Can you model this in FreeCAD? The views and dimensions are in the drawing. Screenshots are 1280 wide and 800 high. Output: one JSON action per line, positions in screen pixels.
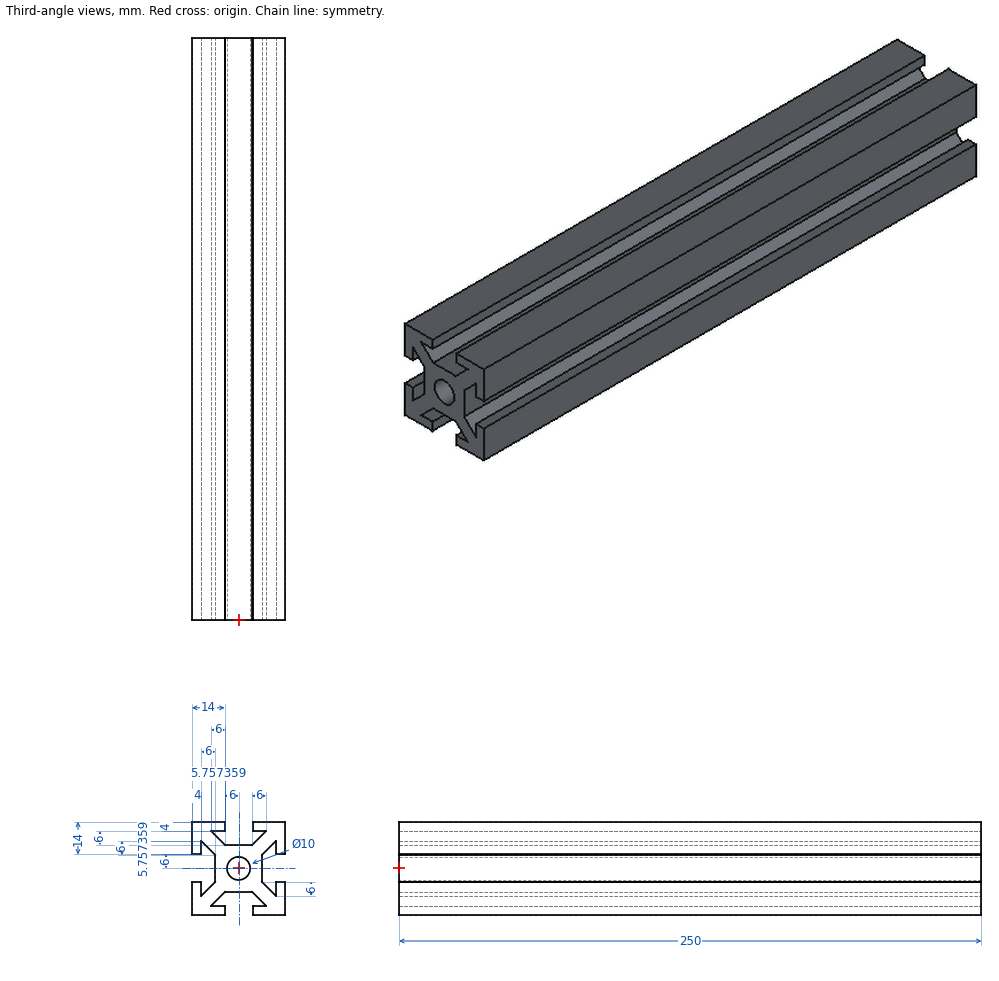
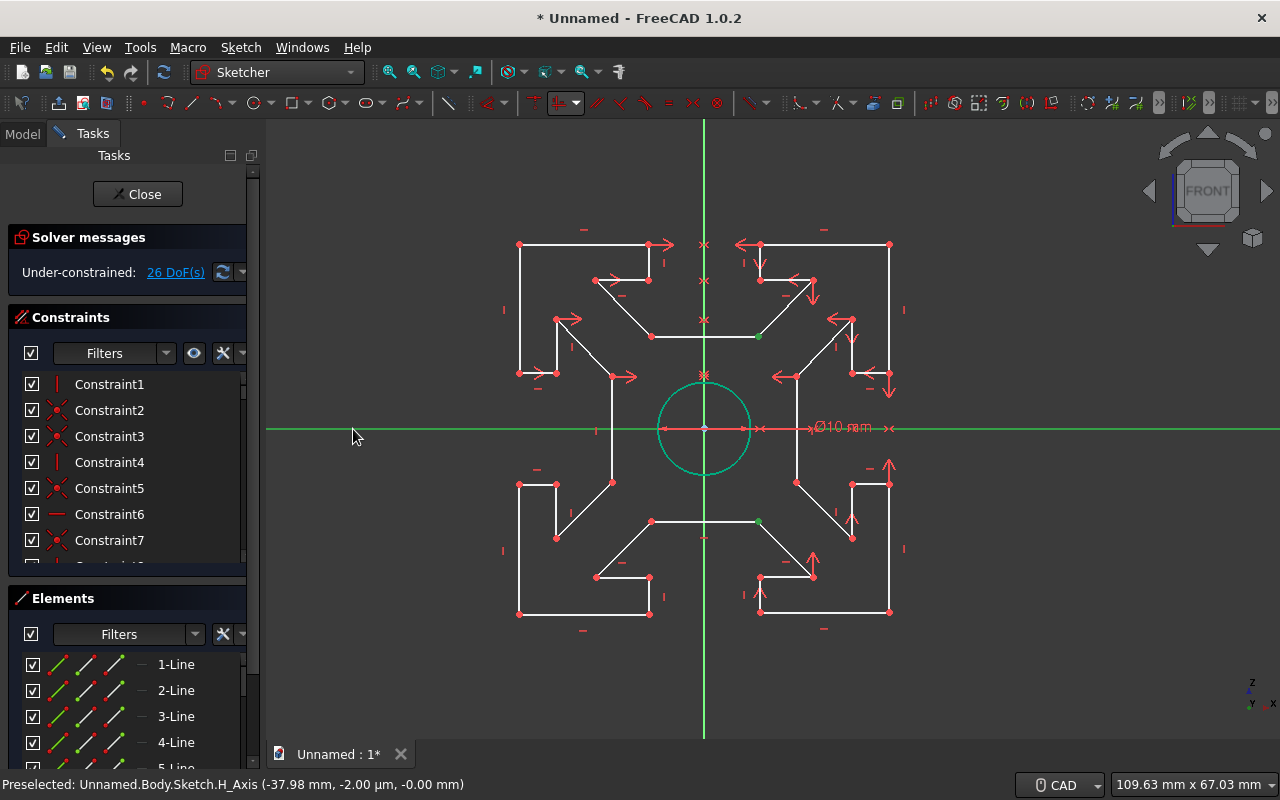
{"action": "left_click", "coordinate": [694, 104]}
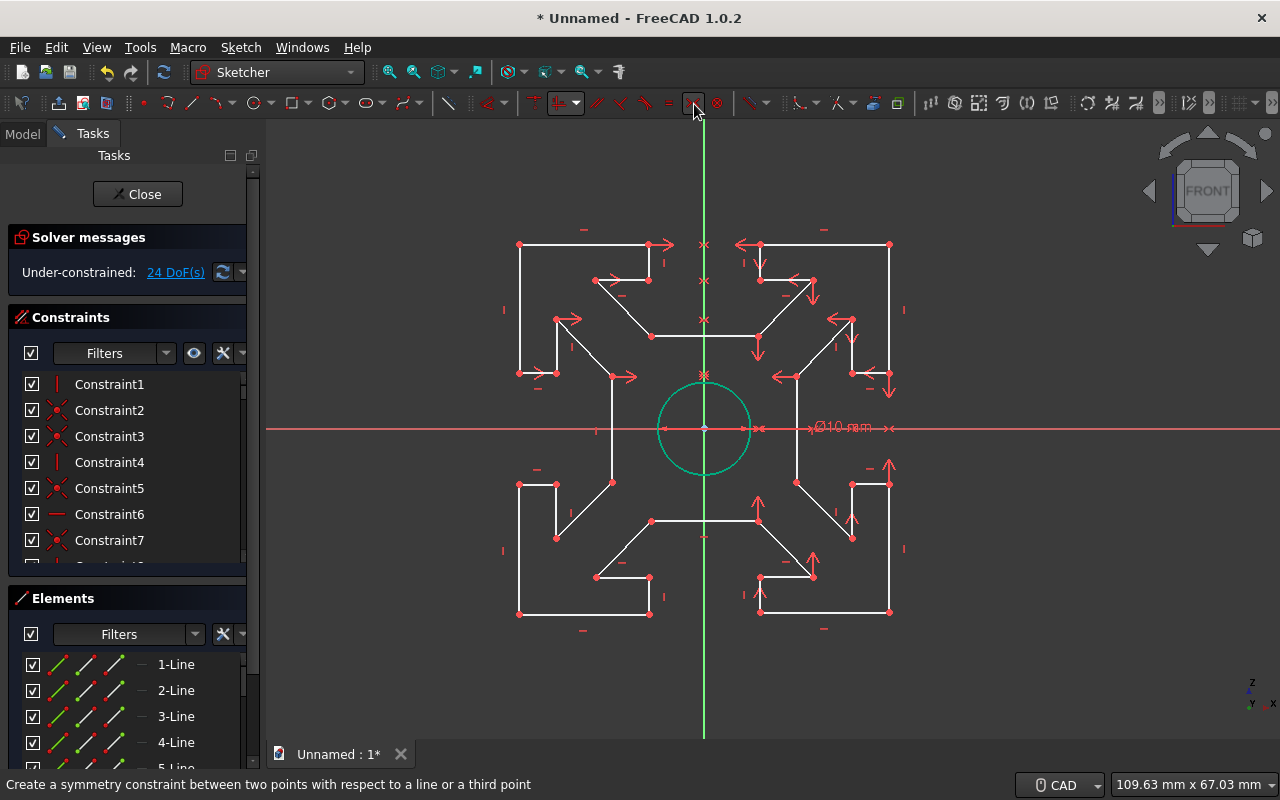
{"action": "left_click", "coordinate": [596, 280]}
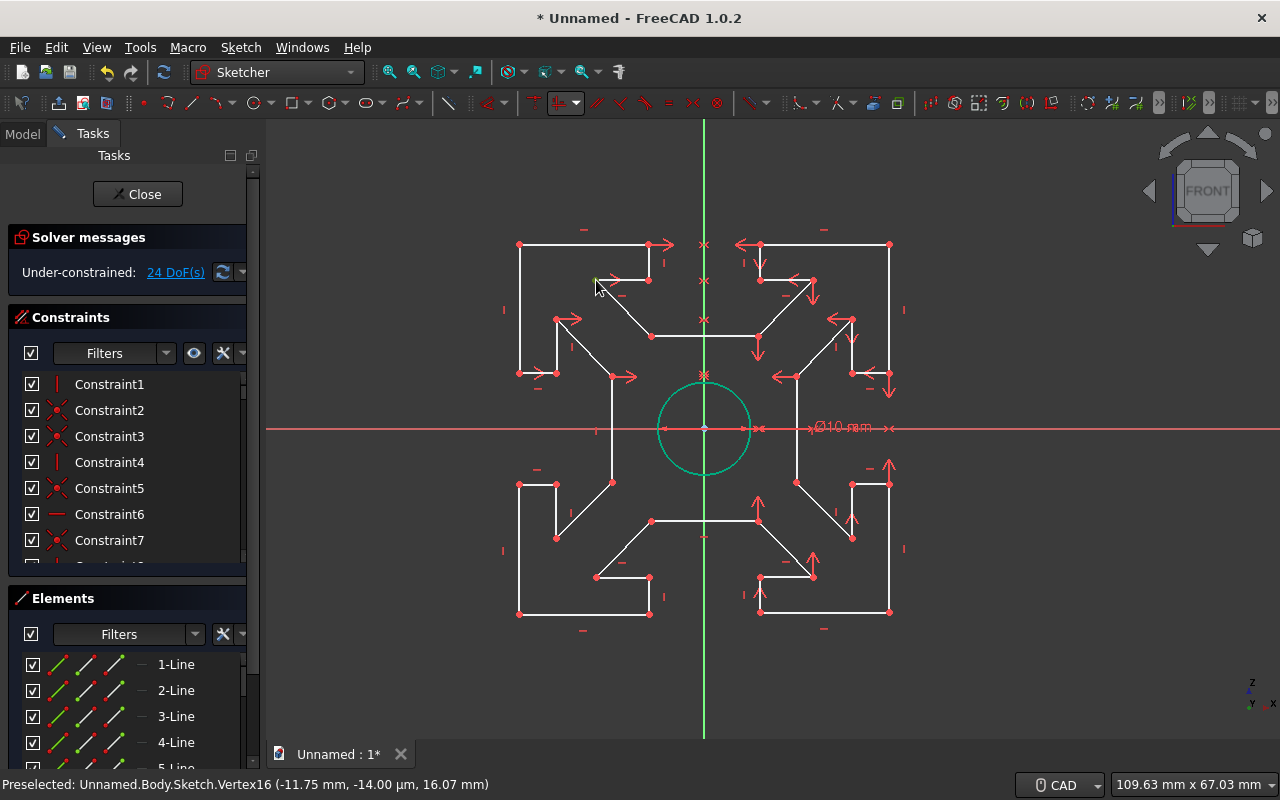
{"action": "left_click", "coordinate": [596, 578]}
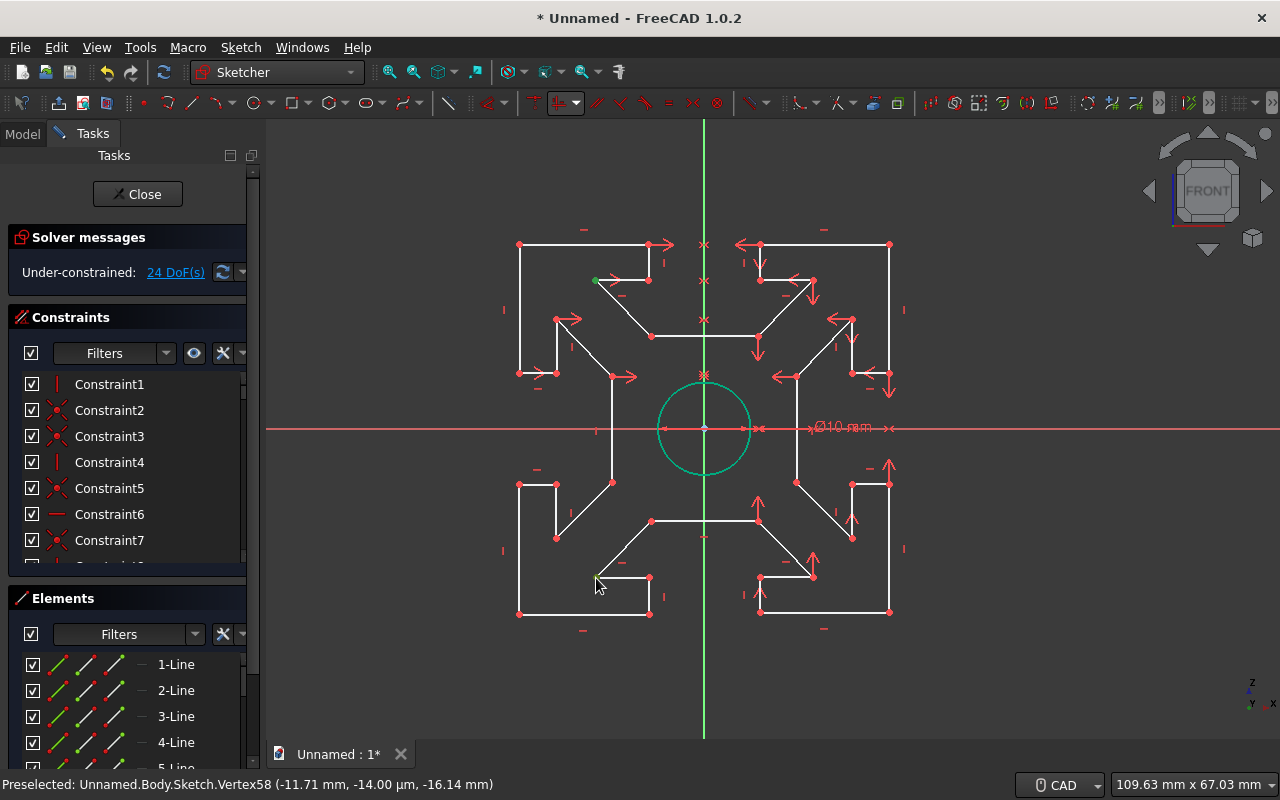
{"action": "left_click", "coordinate": [353, 429]}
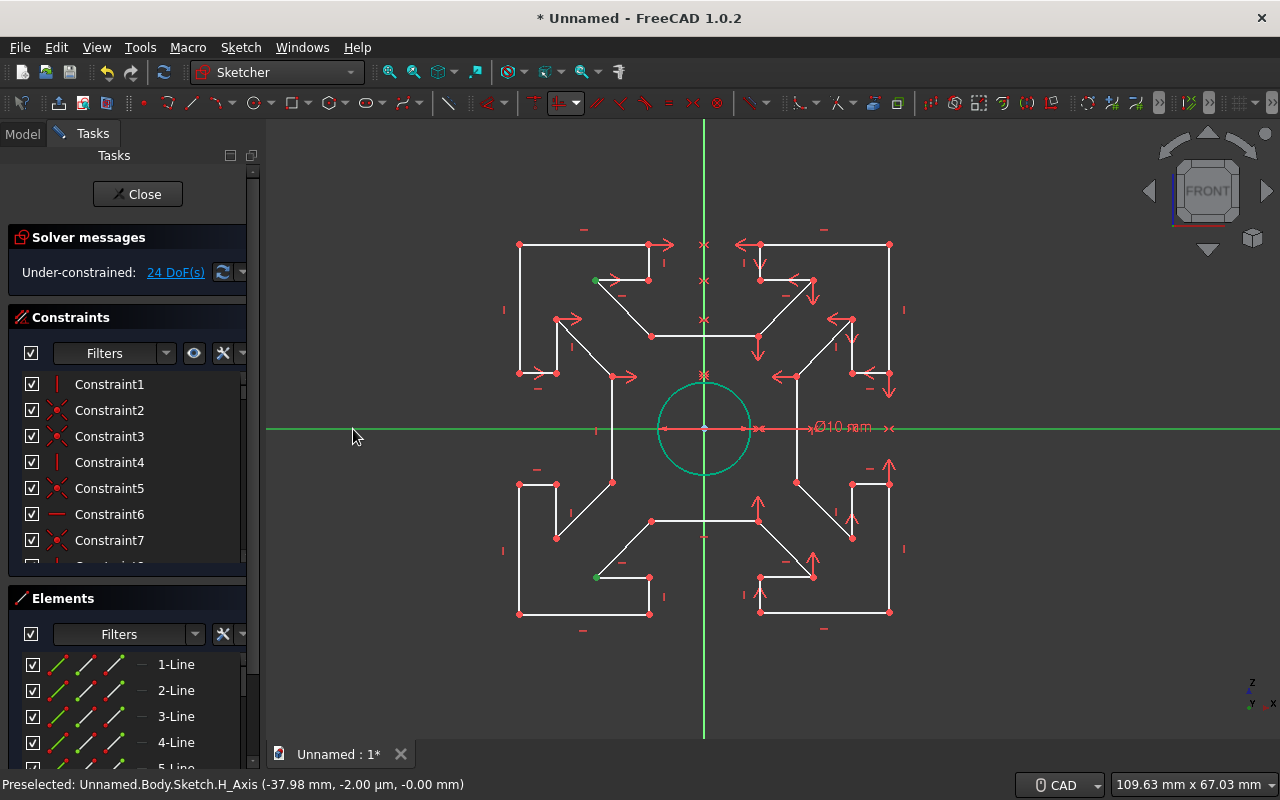
{"action": "left_click", "coordinate": [694, 104]}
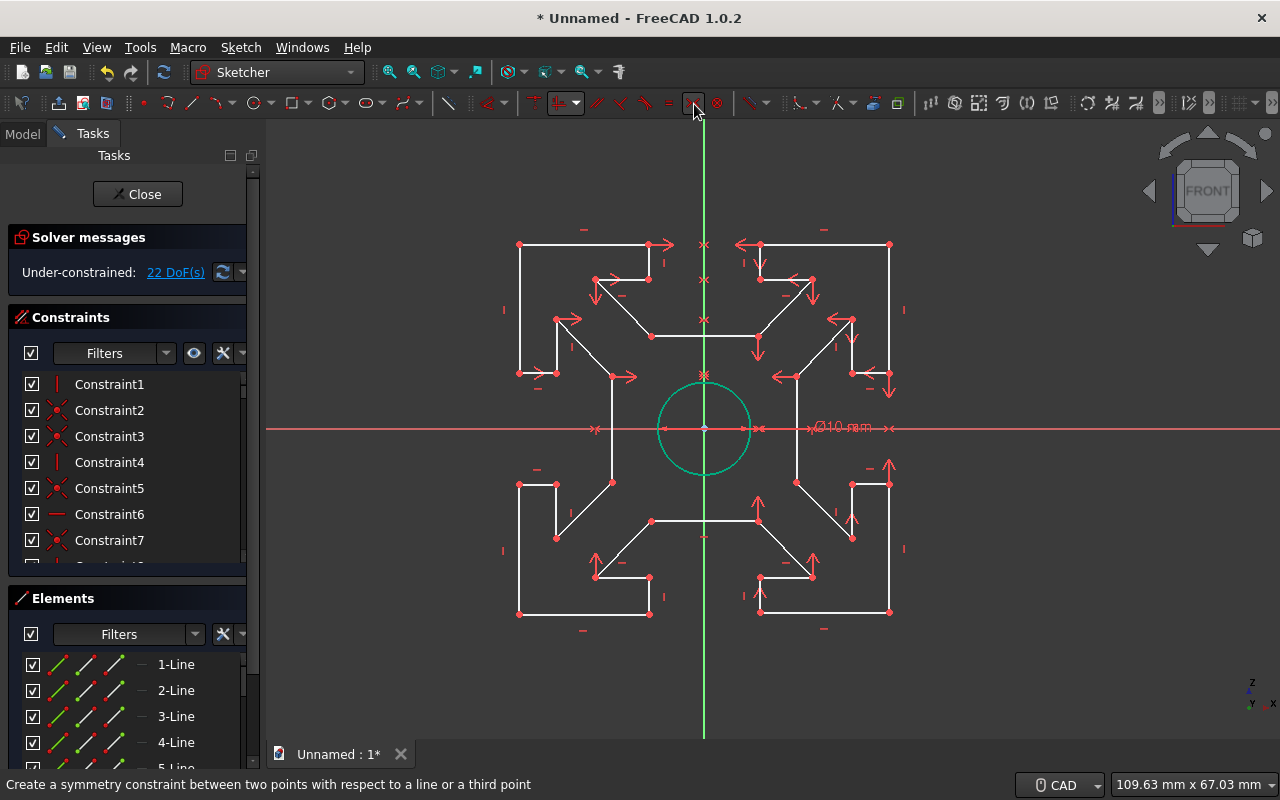
{"action": "left_click", "coordinate": [649, 245]}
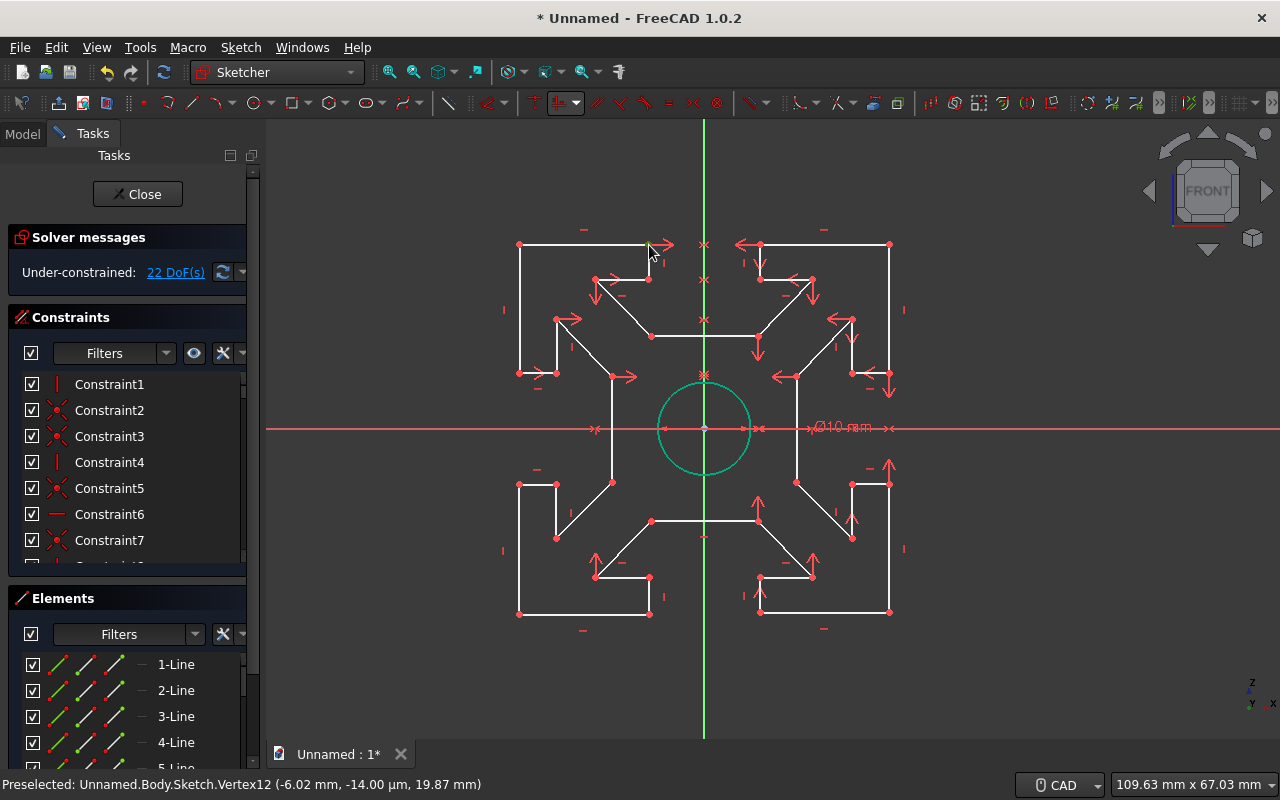
{"action": "left_click", "coordinate": [649, 615]}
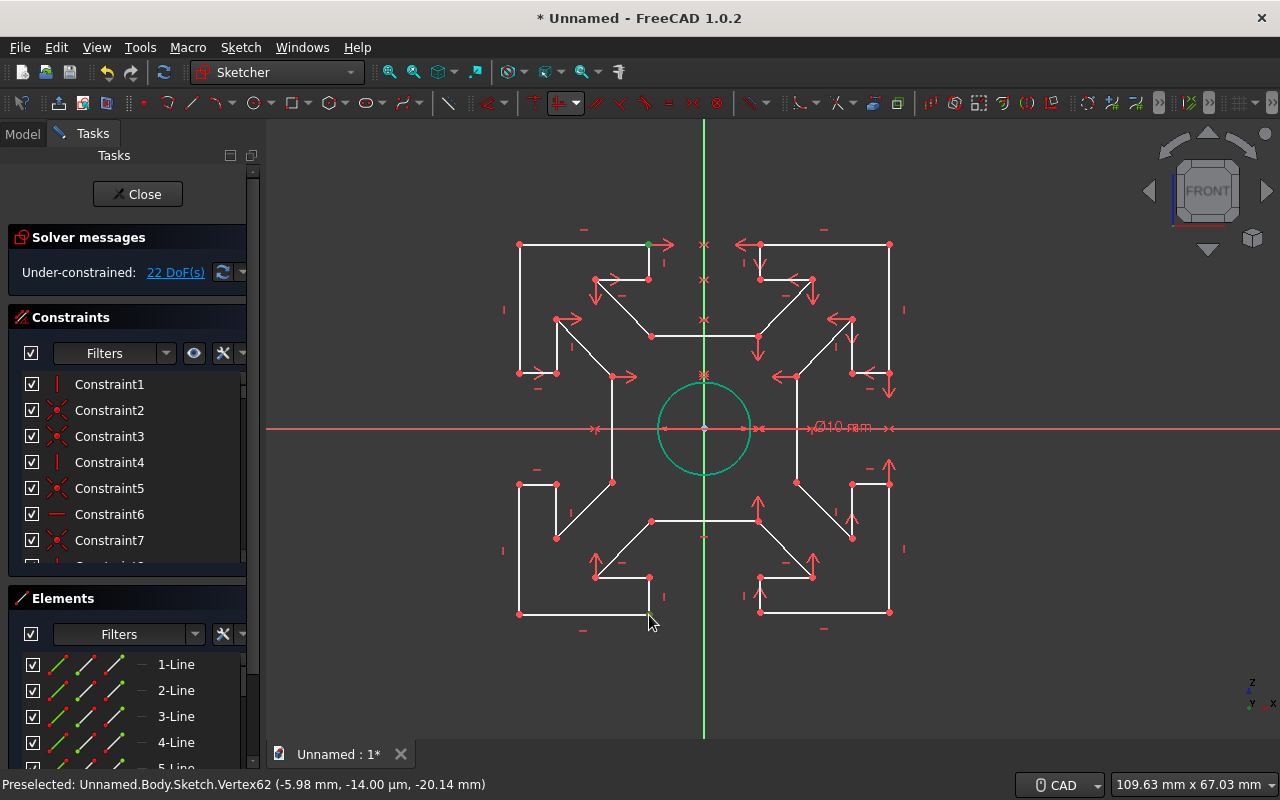
{"action": "left_click", "coordinate": [353, 429]}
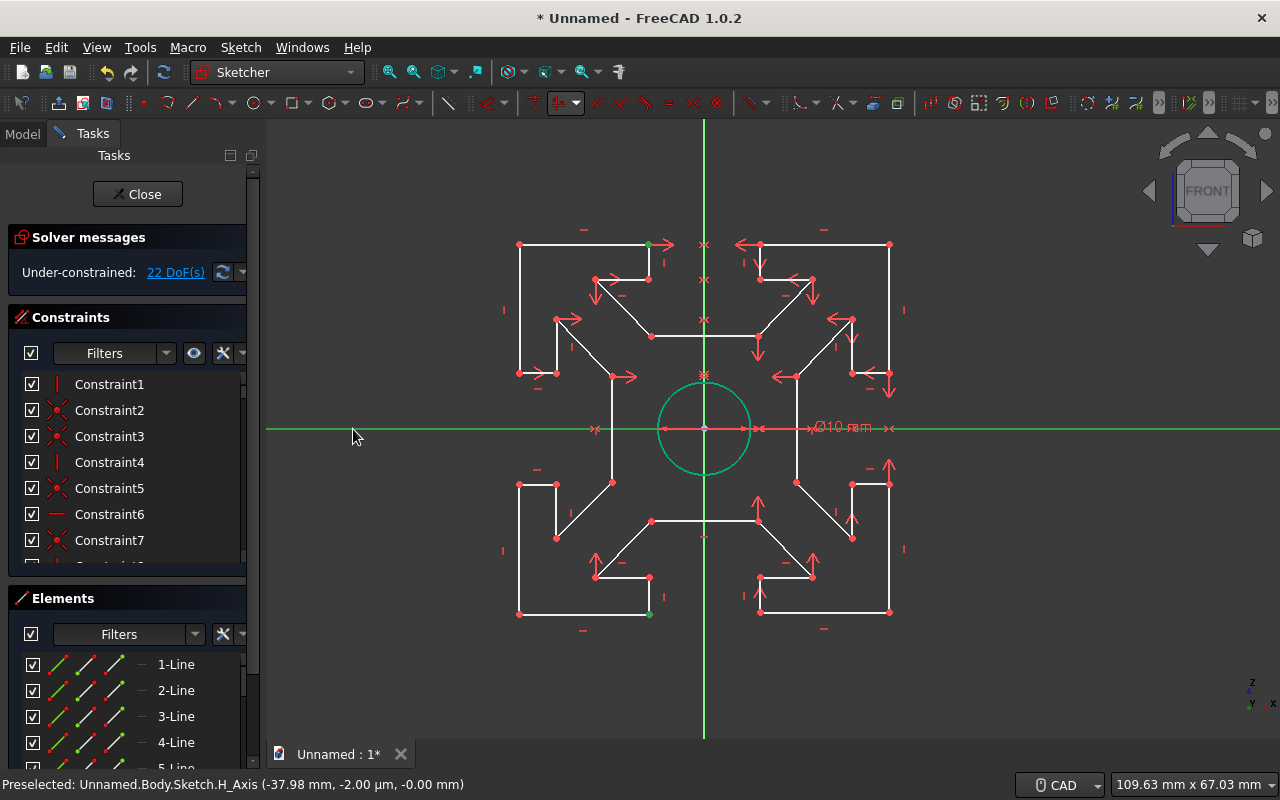
{"action": "left_click", "coordinate": [694, 104]}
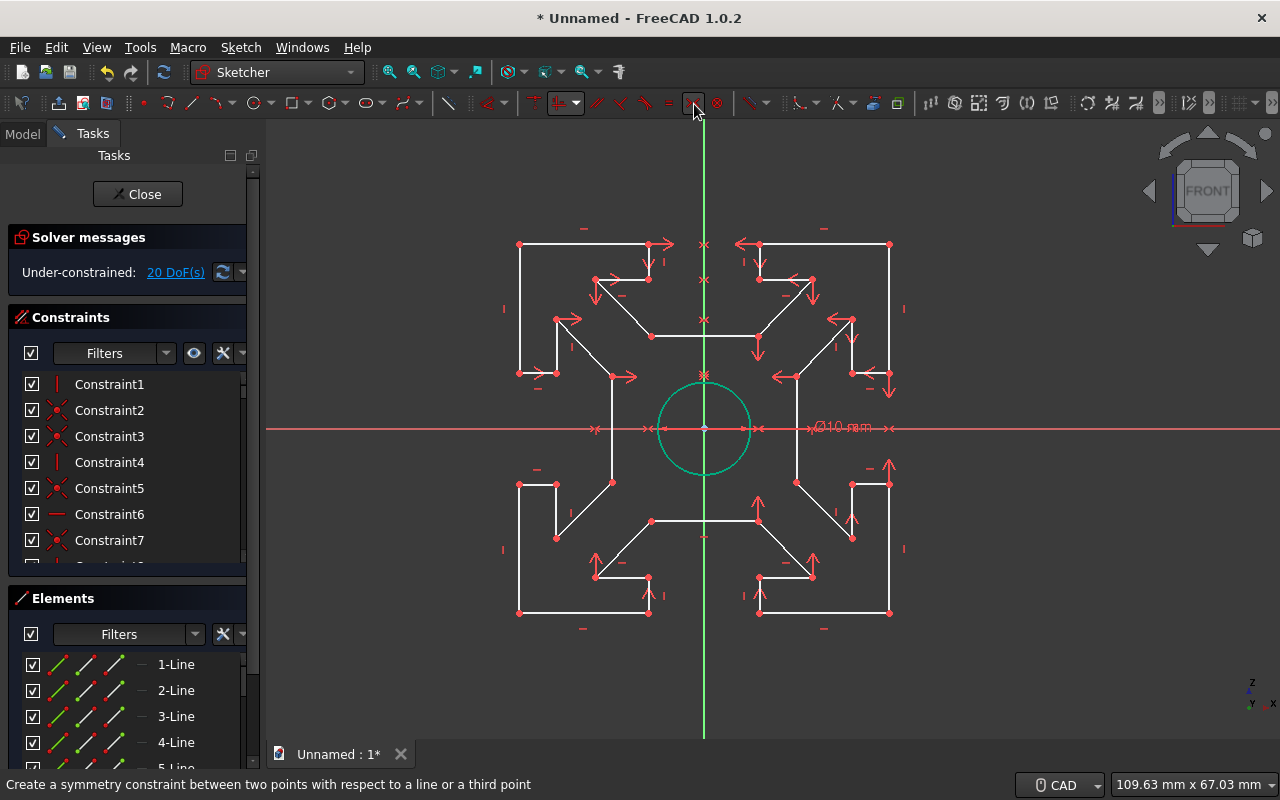
{"action": "left_click", "coordinate": [520, 373]}